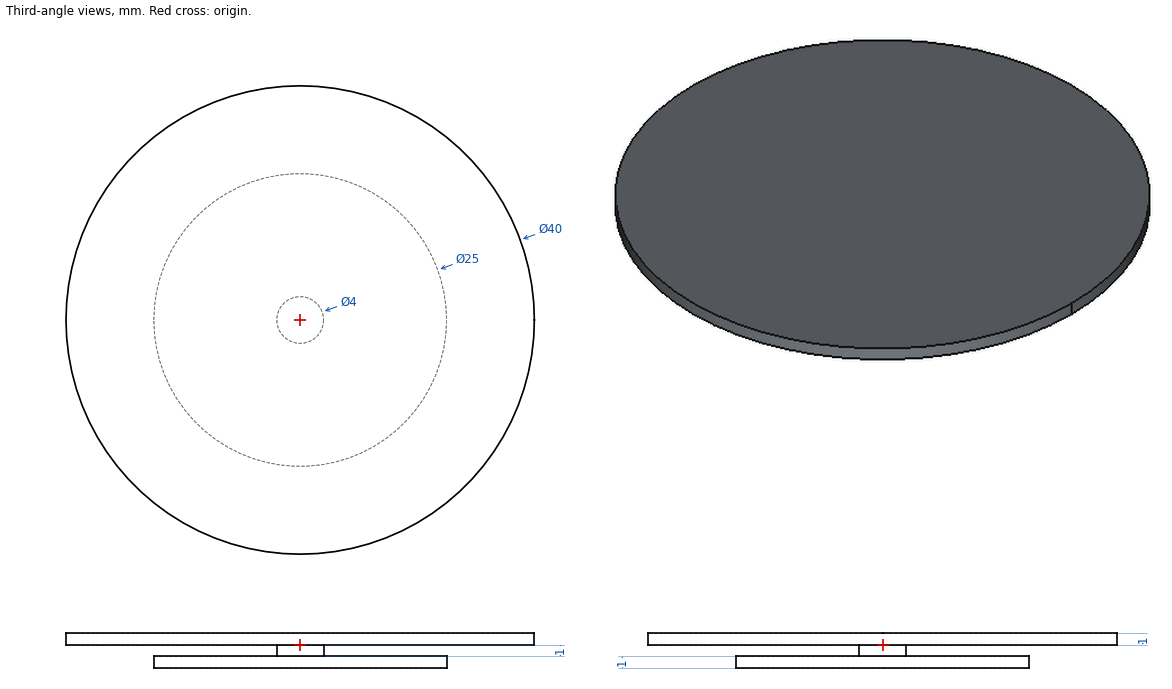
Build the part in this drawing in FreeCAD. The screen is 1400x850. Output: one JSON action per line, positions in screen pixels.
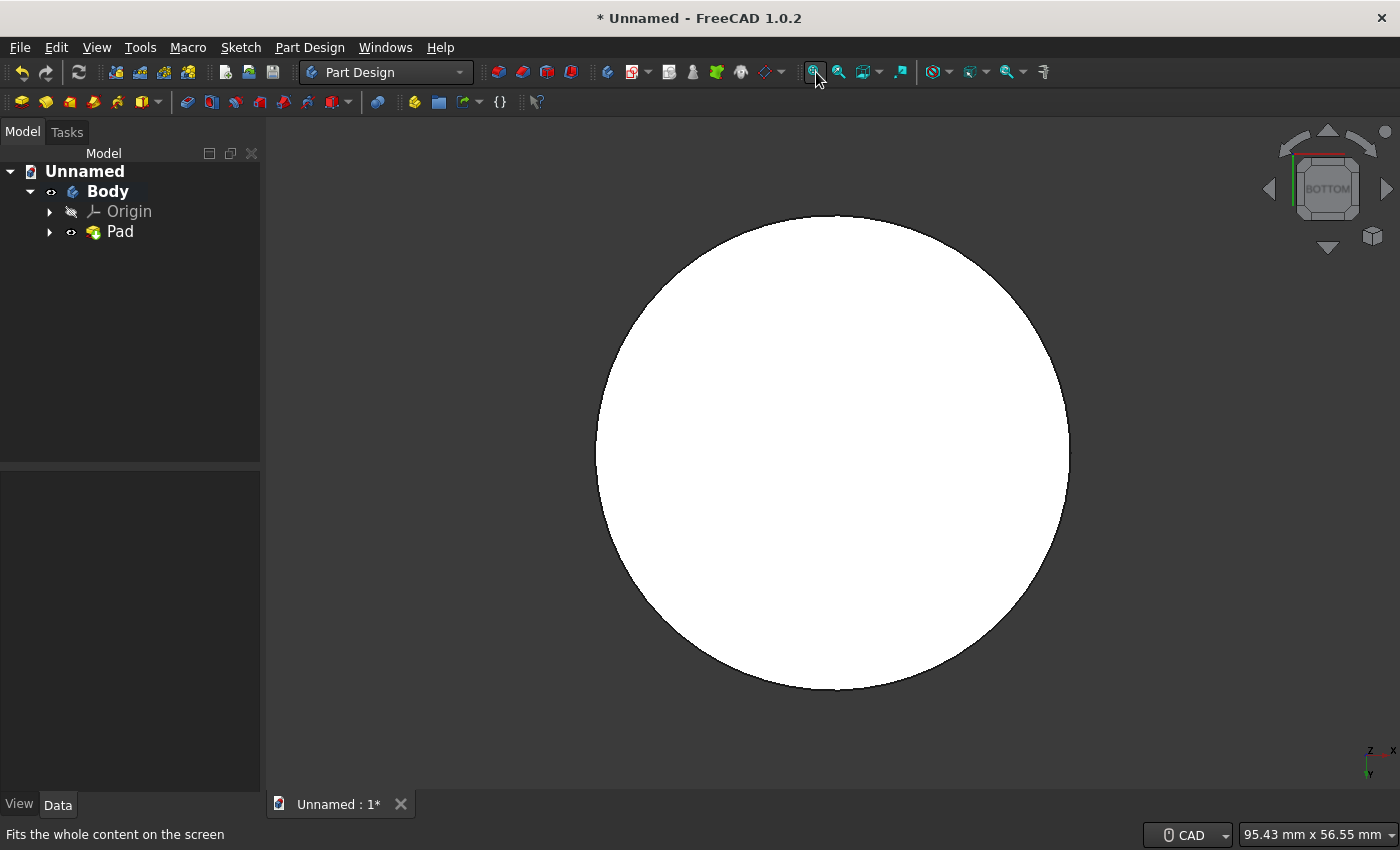
{"action": "left_click", "coordinate": [833, 452]}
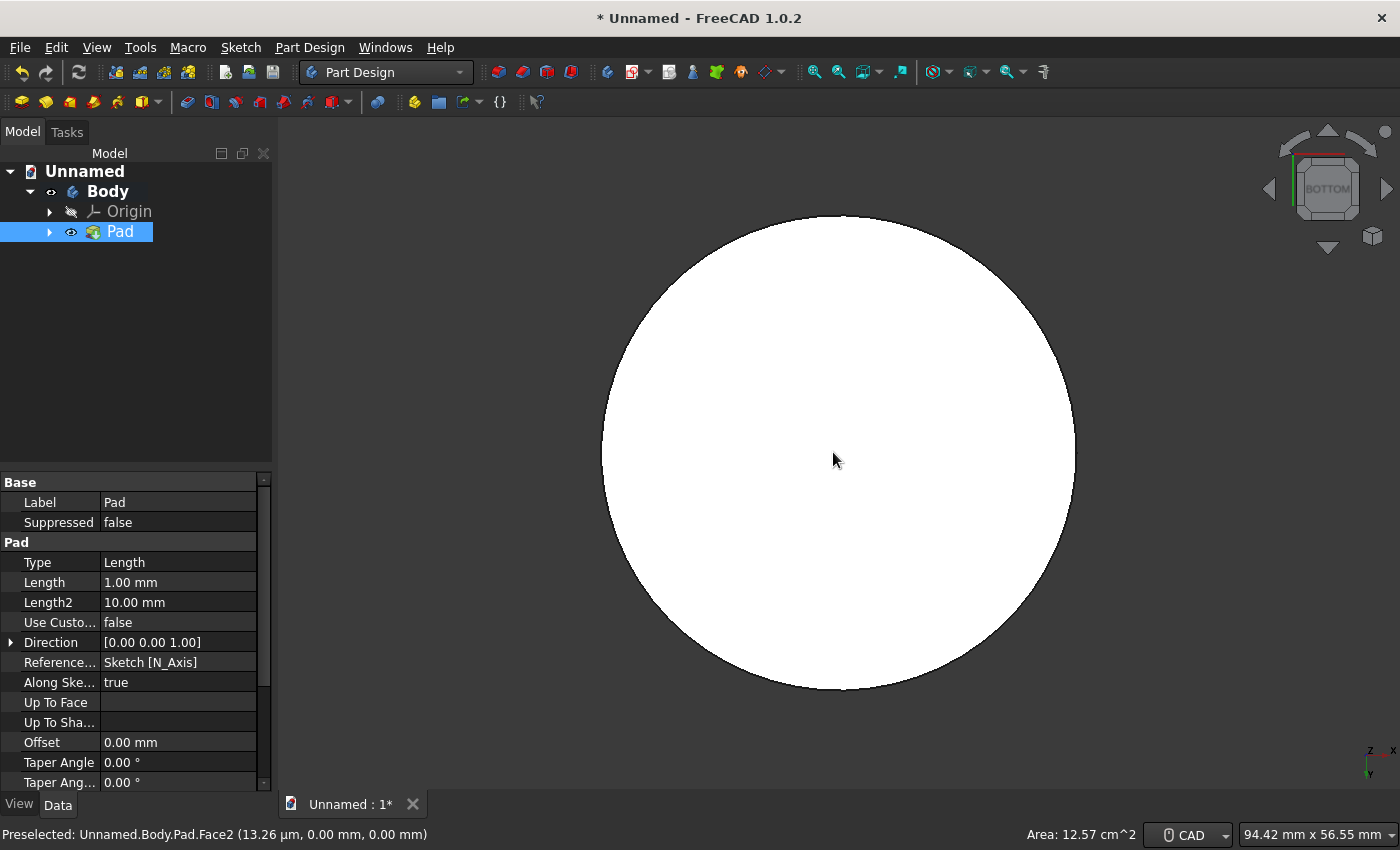
{"action": "left_click", "coordinate": [632, 72]}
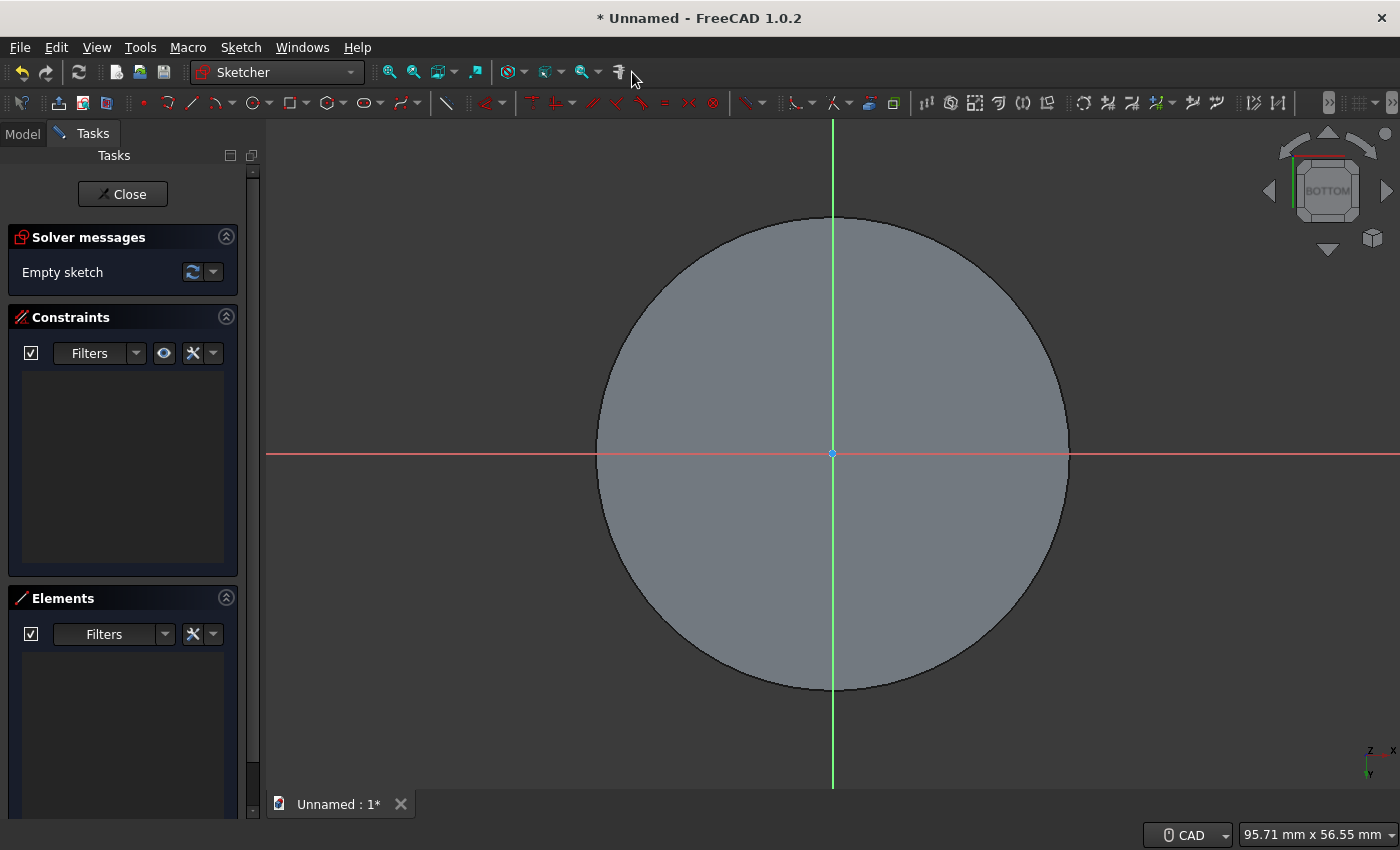
{"action": "scroll", "coordinate": [841, 454], "scroll_direction": "up", "scroll_amount": 11}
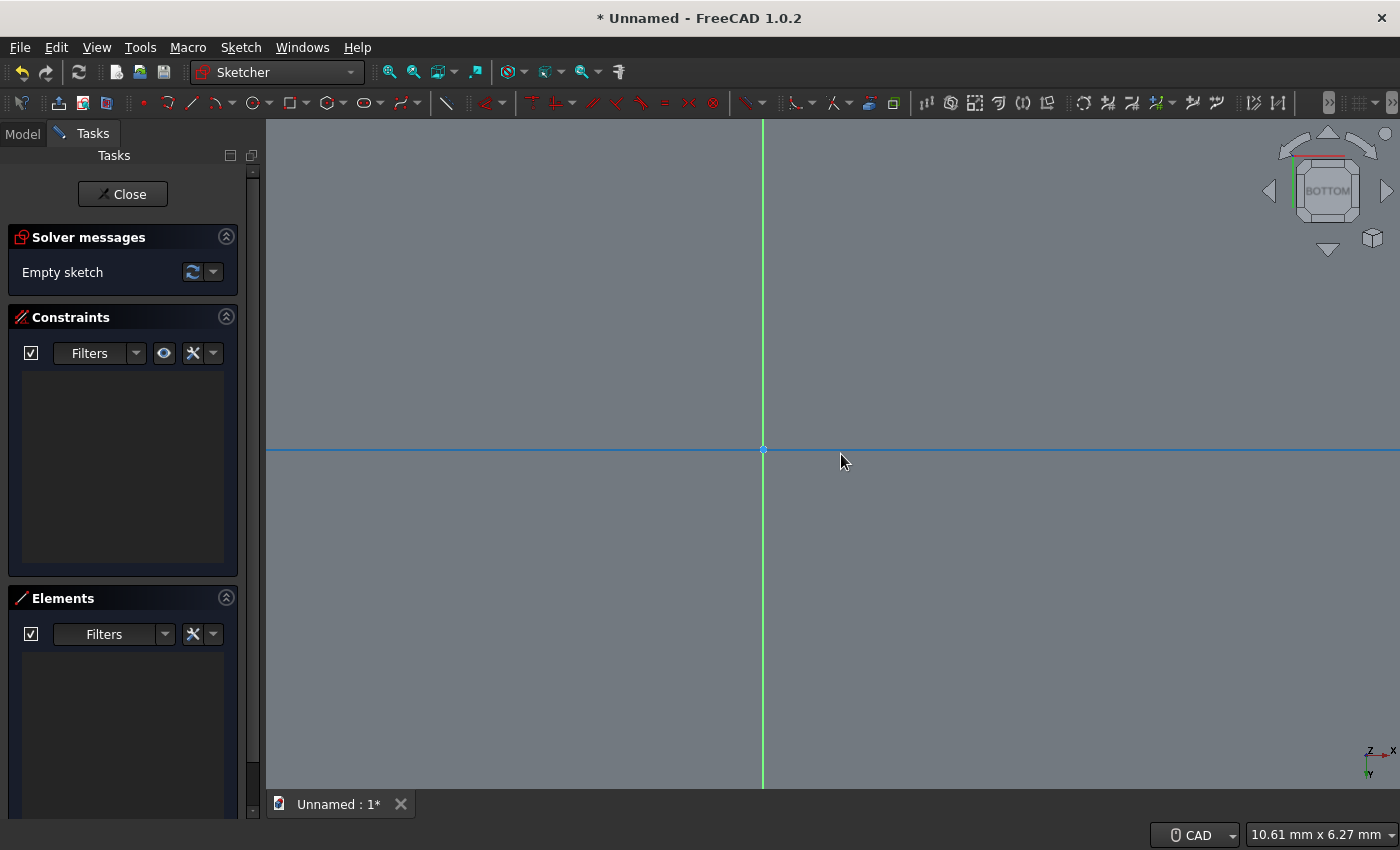
{"action": "key", "text": "g c"}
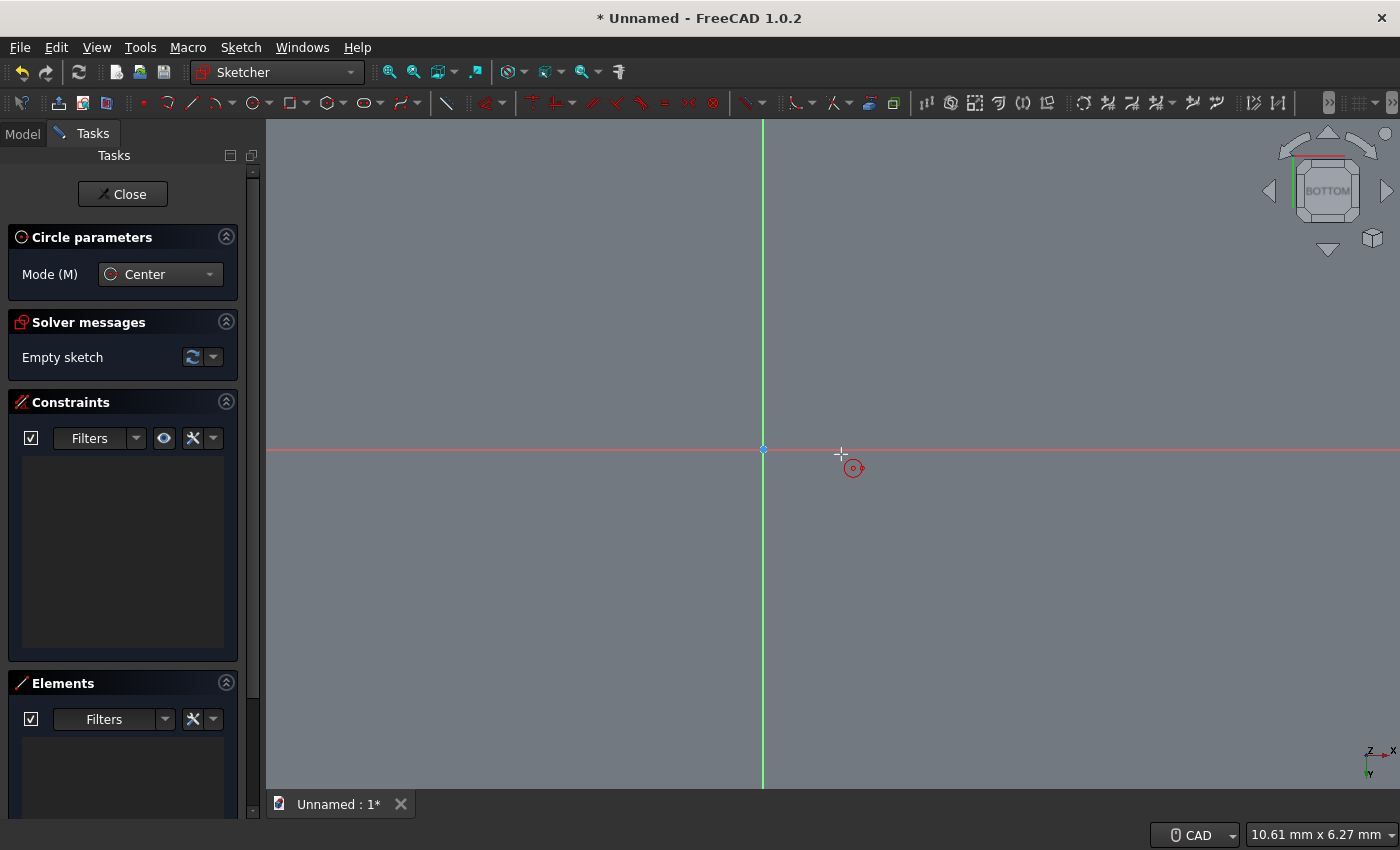
{"action": "left_click", "coordinate": [763, 450]}
{"action": "left_click", "coordinate": [915, 299]}
{"action": "key", "text": "Escape"}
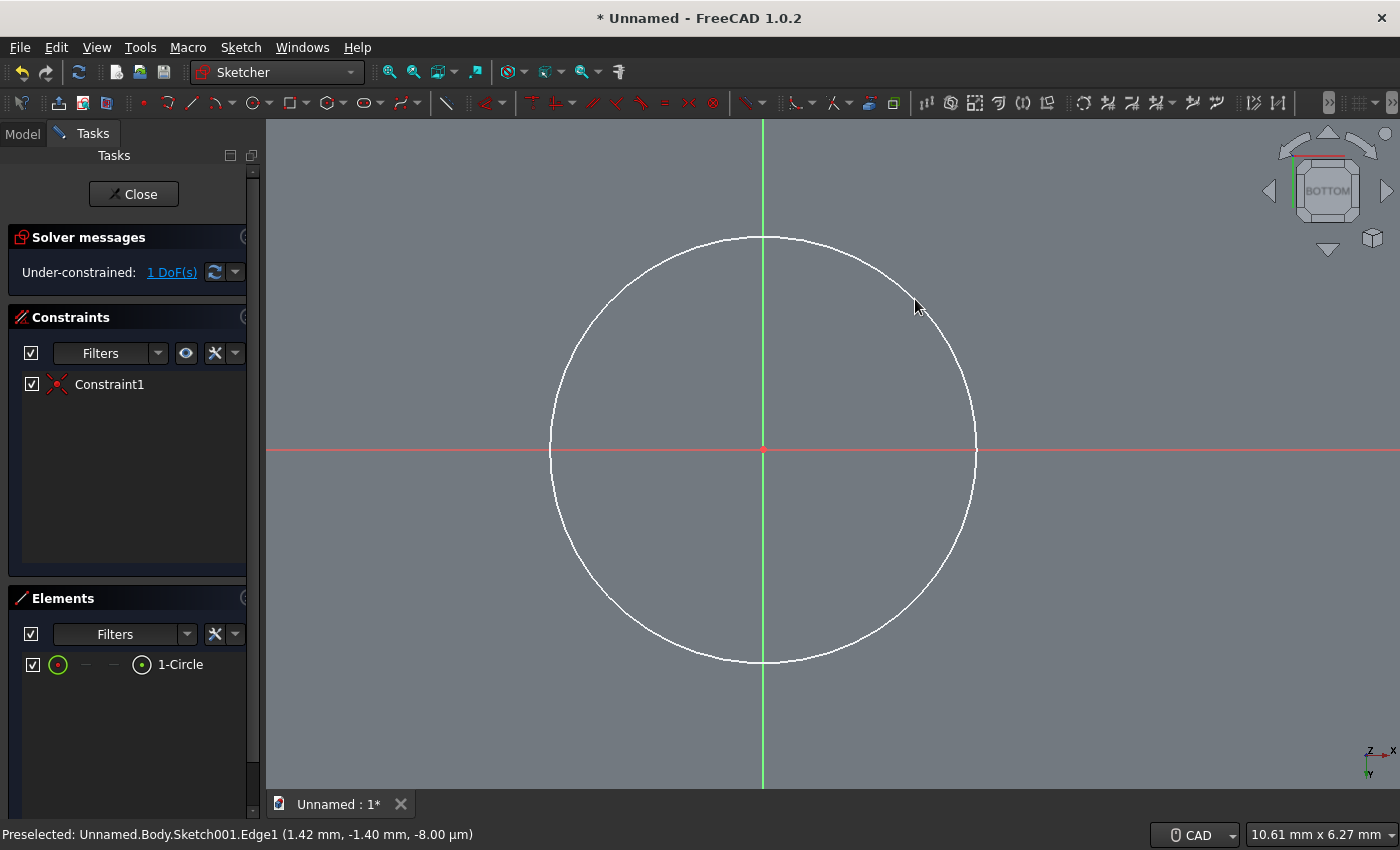
{"action": "left_click", "coordinate": [486, 104]}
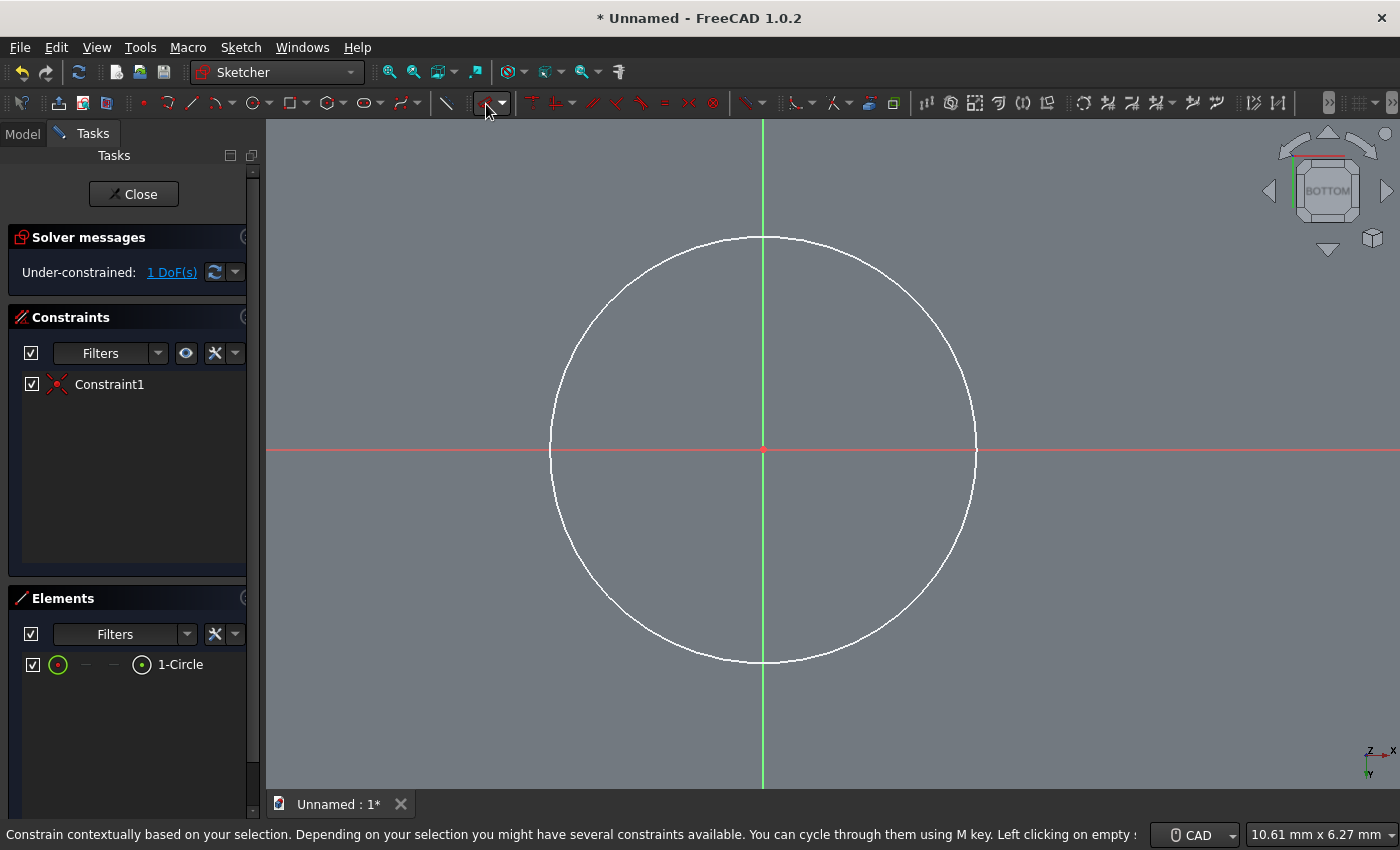
{"action": "left_click", "coordinate": [914, 299]}
{"action": "left_click", "coordinate": [937, 276]}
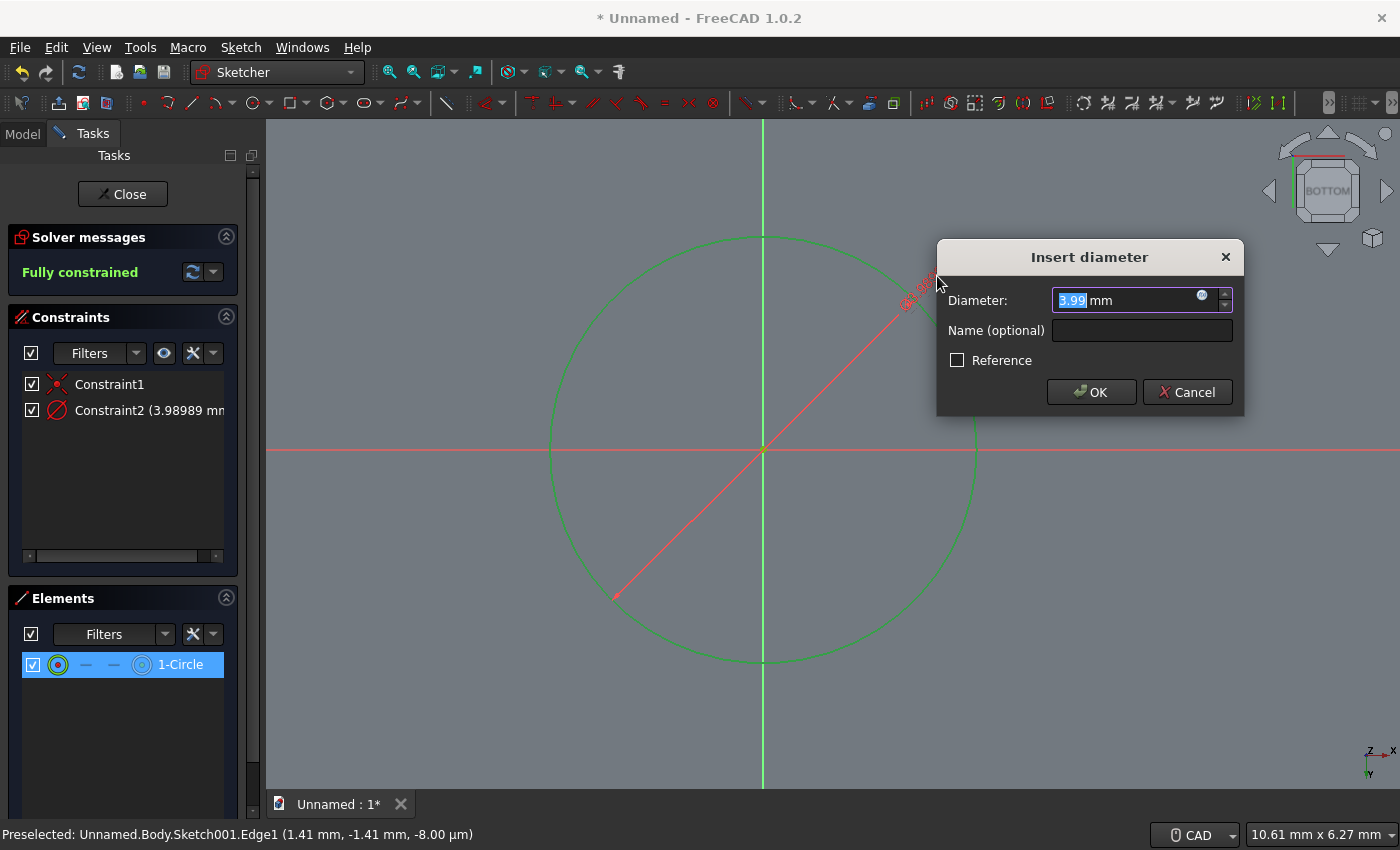
{"action": "type", "text": "4"}
{"action": "key", "text": "Return"}
{"action": "key", "text": "Escape"}